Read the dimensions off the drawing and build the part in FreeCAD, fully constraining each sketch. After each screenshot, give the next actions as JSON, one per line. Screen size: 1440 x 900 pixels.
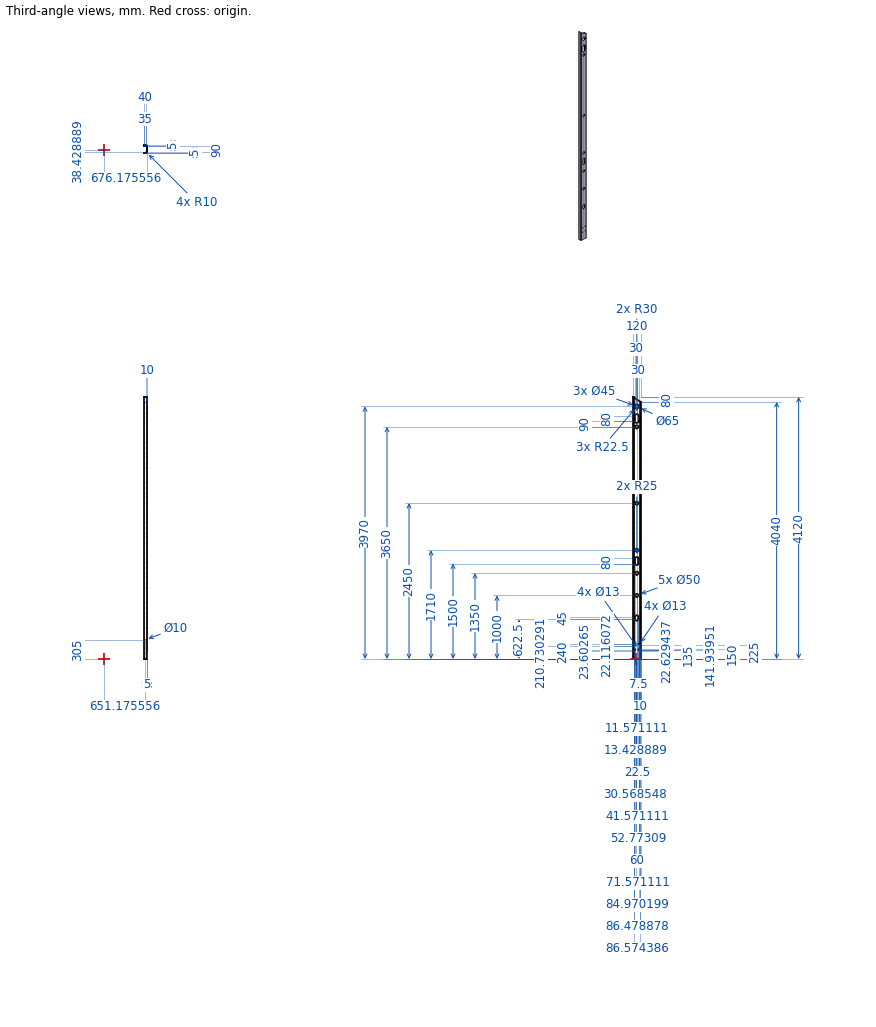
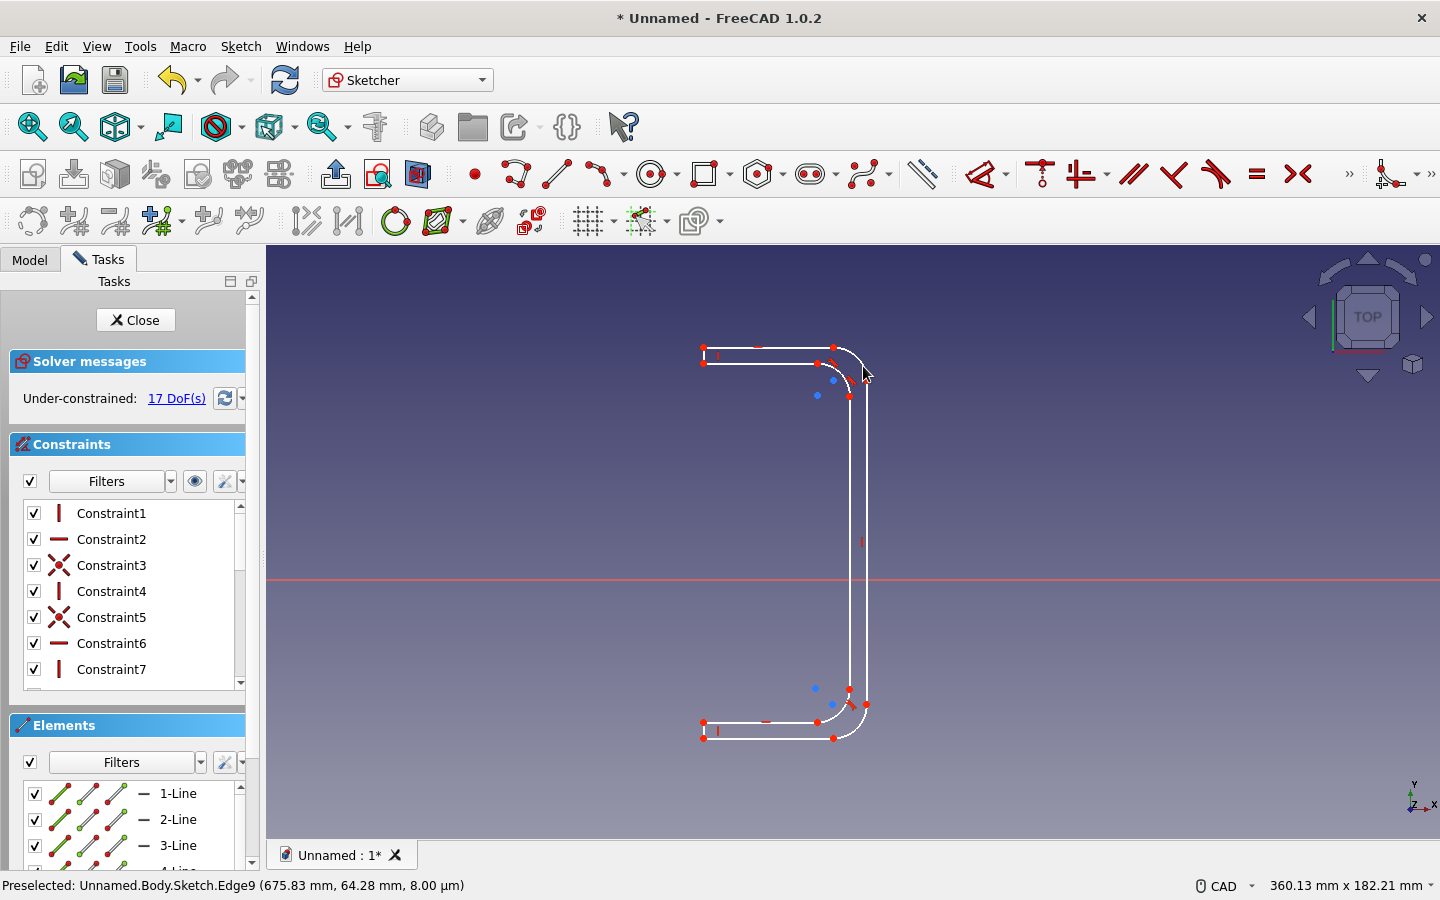
{"action": "left_click", "coordinate": [738, 364]}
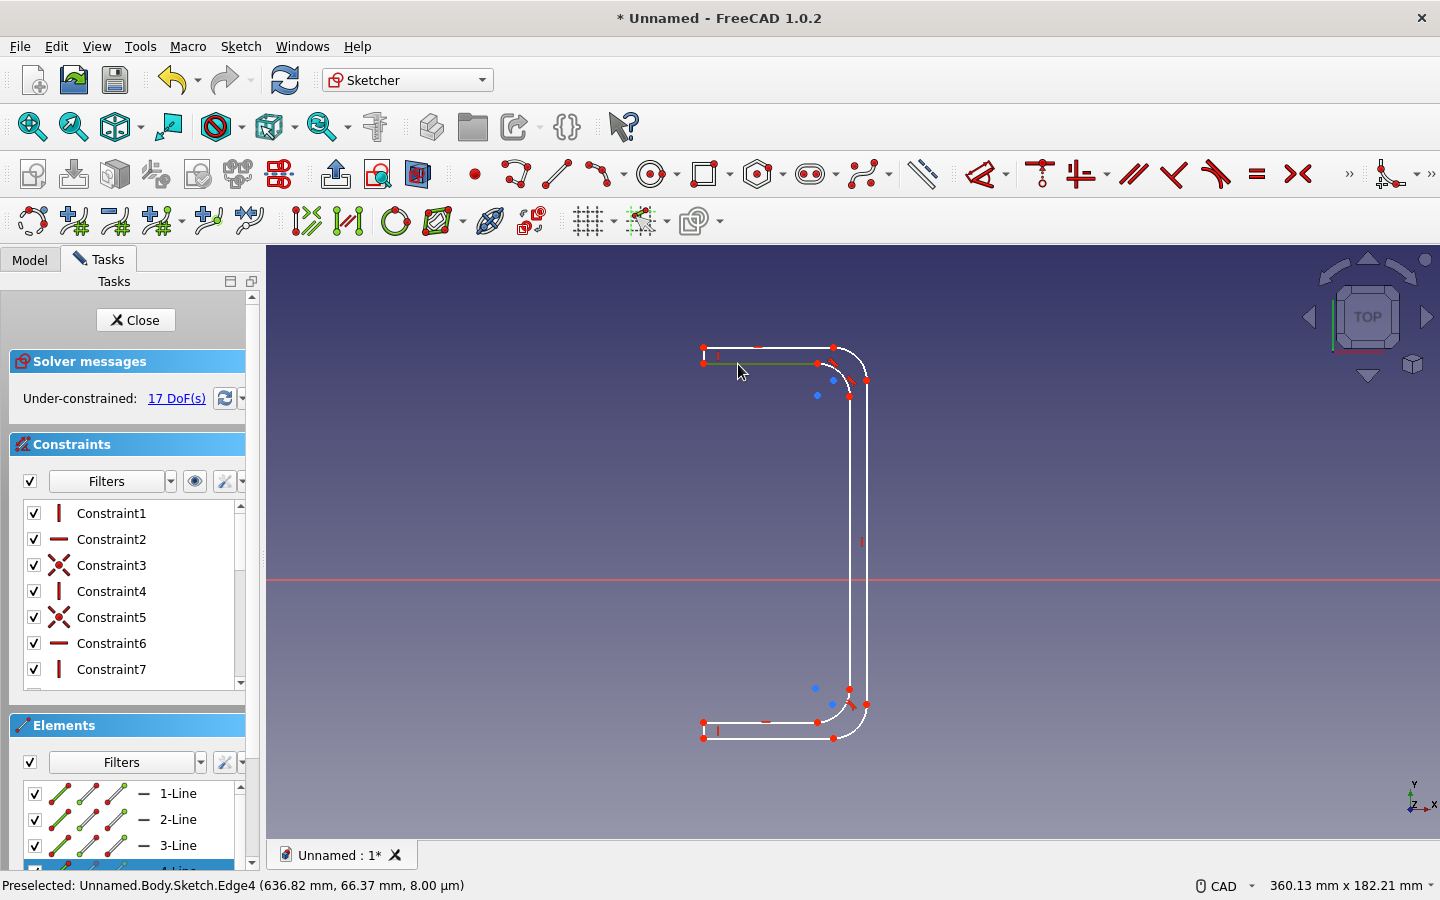
{"action": "left_click", "coordinate": [841, 373]}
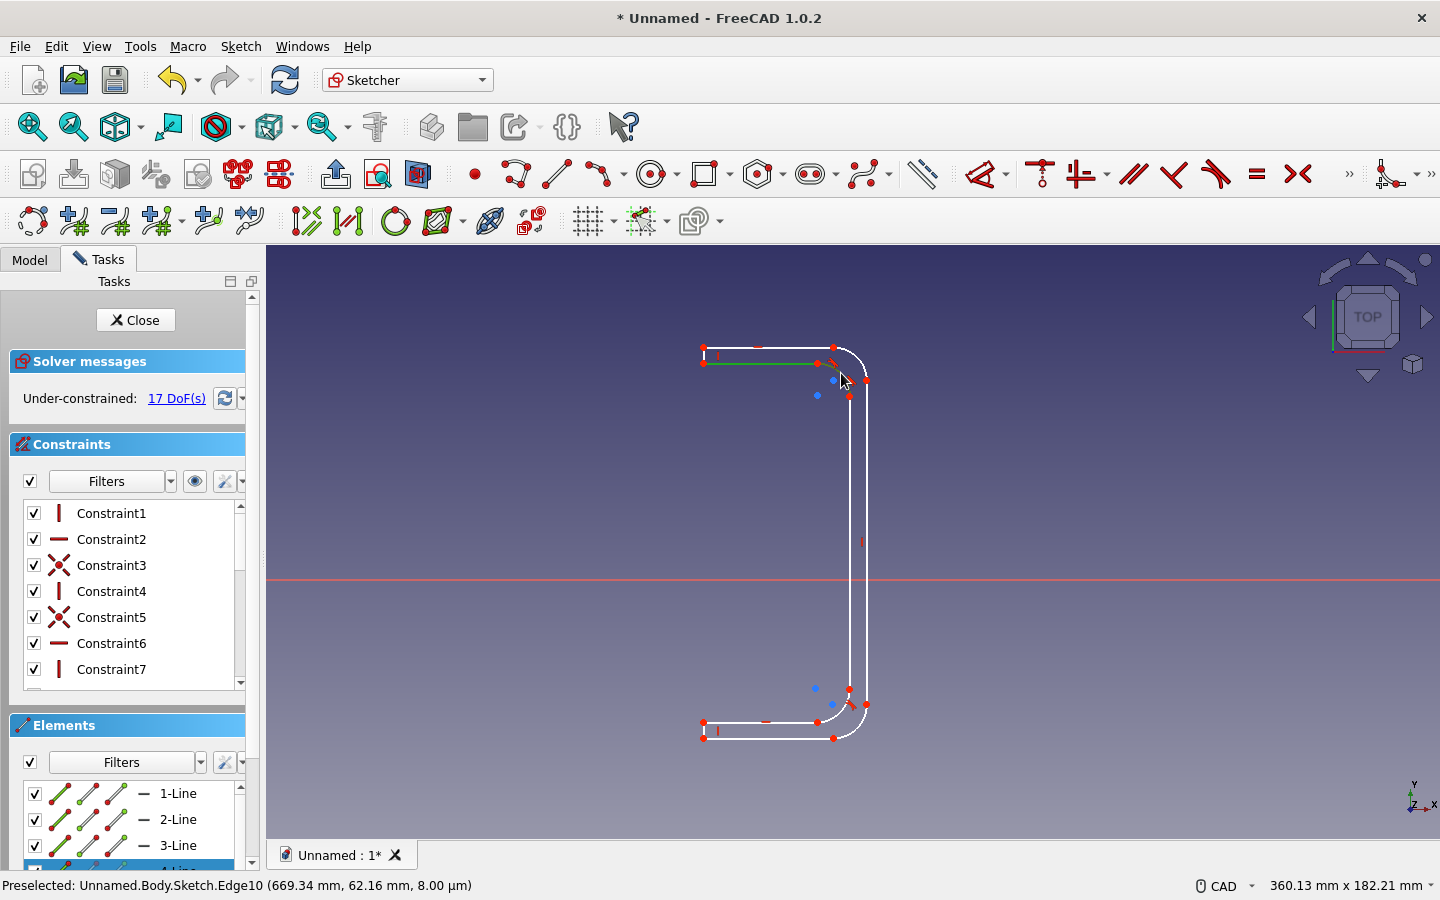
{"action": "key", "text": "t"}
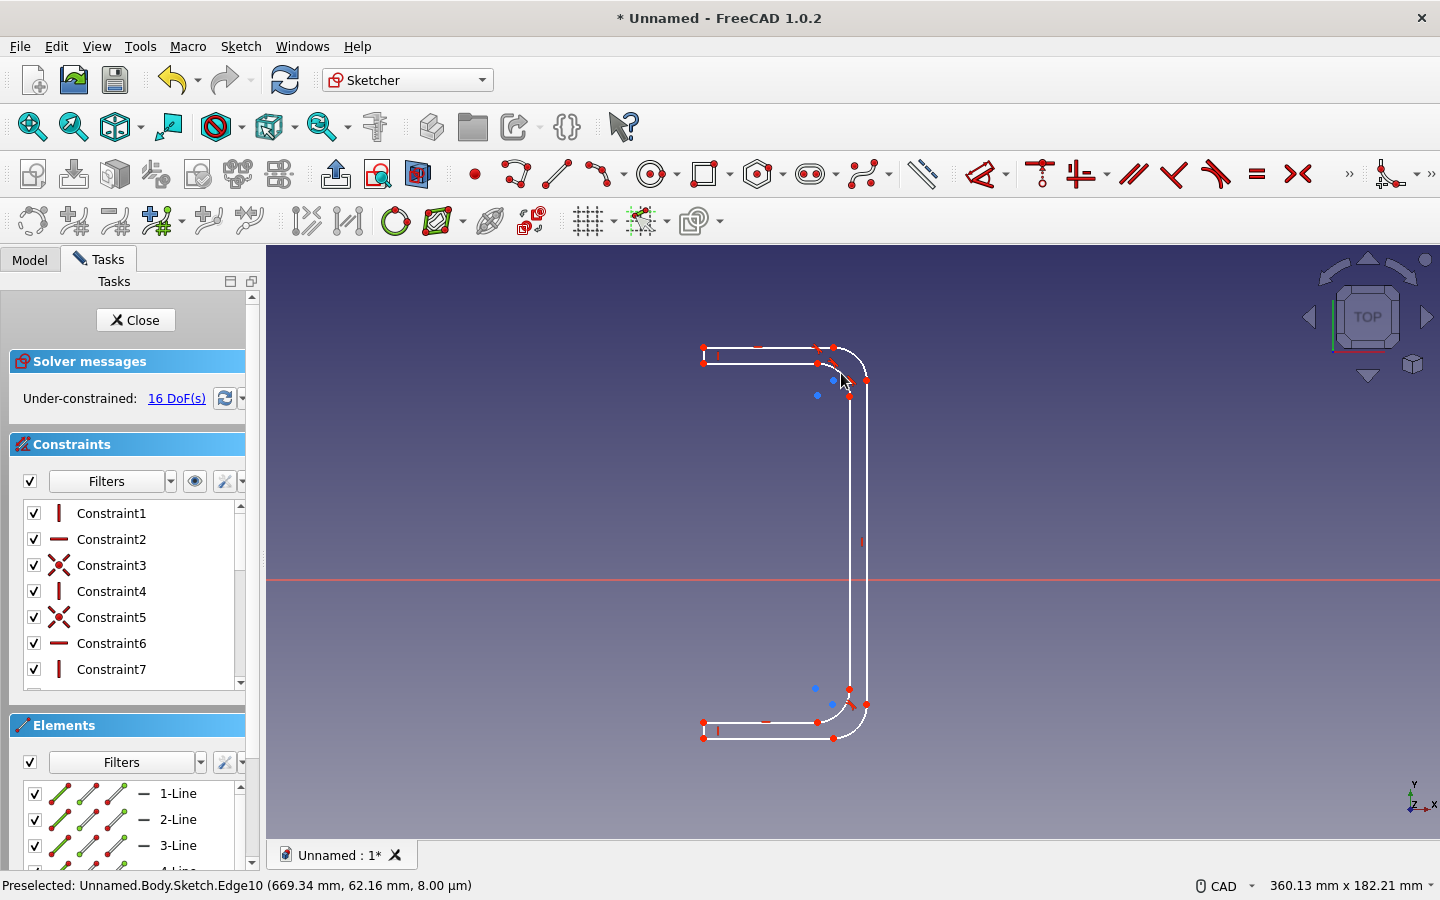
{"action": "left_click", "coordinate": [850, 485]}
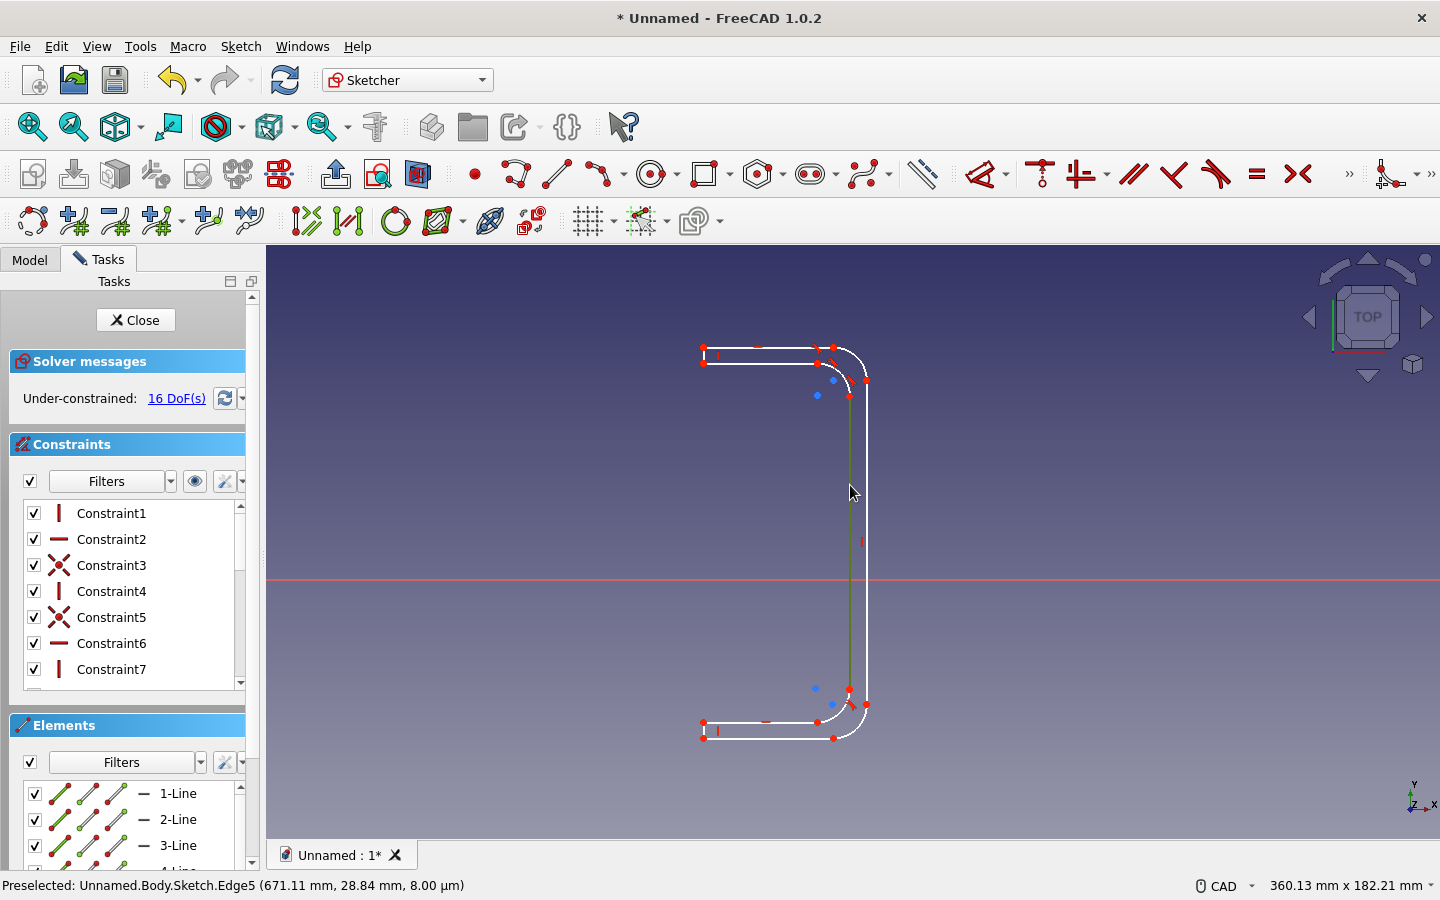
{"action": "left_click", "coordinate": [841, 373]}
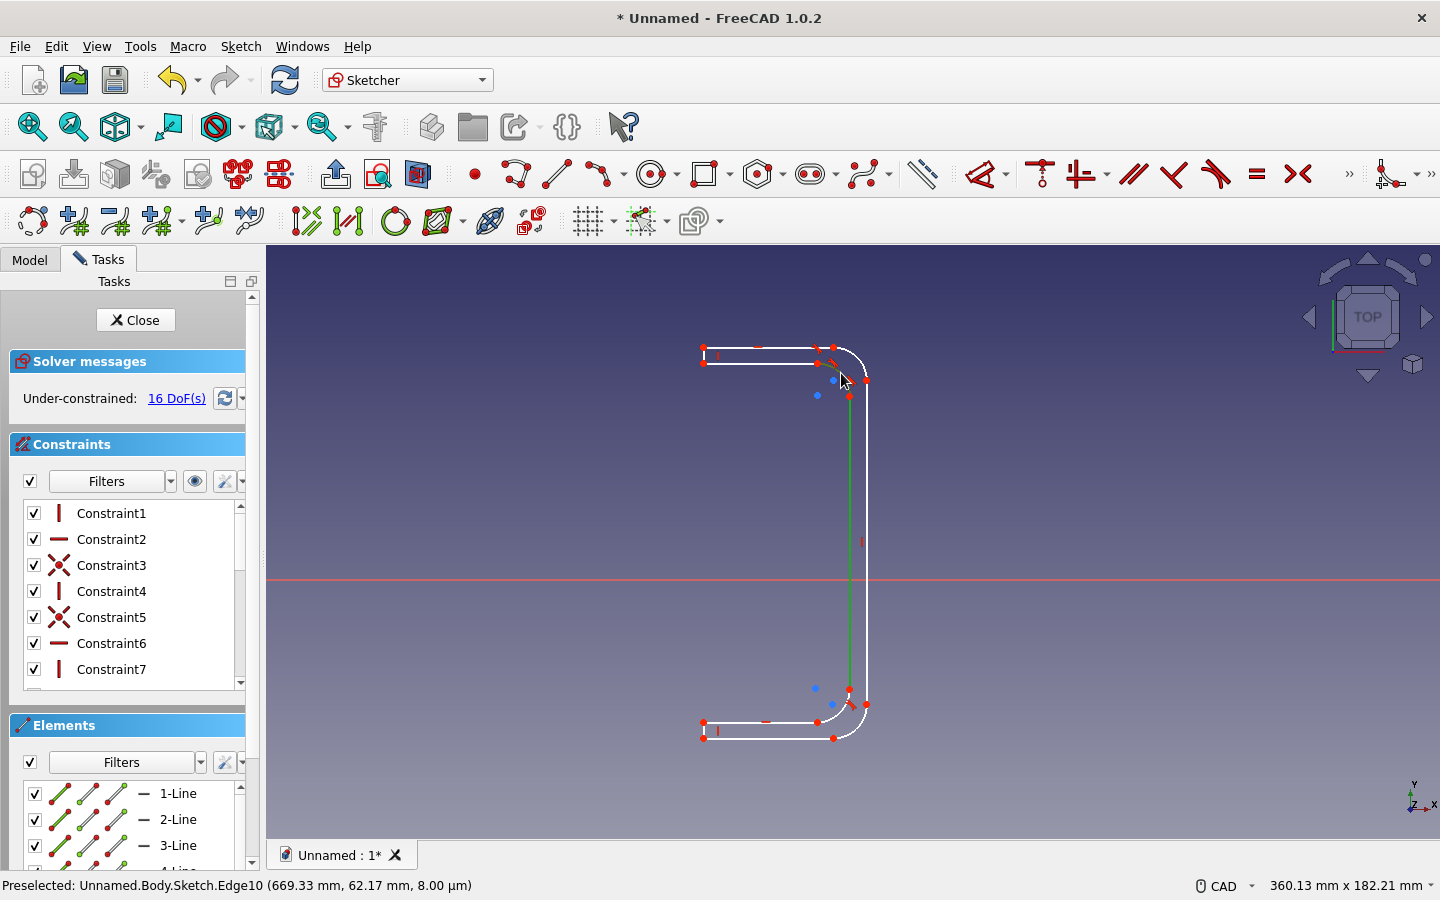
{"action": "key", "text": "t"}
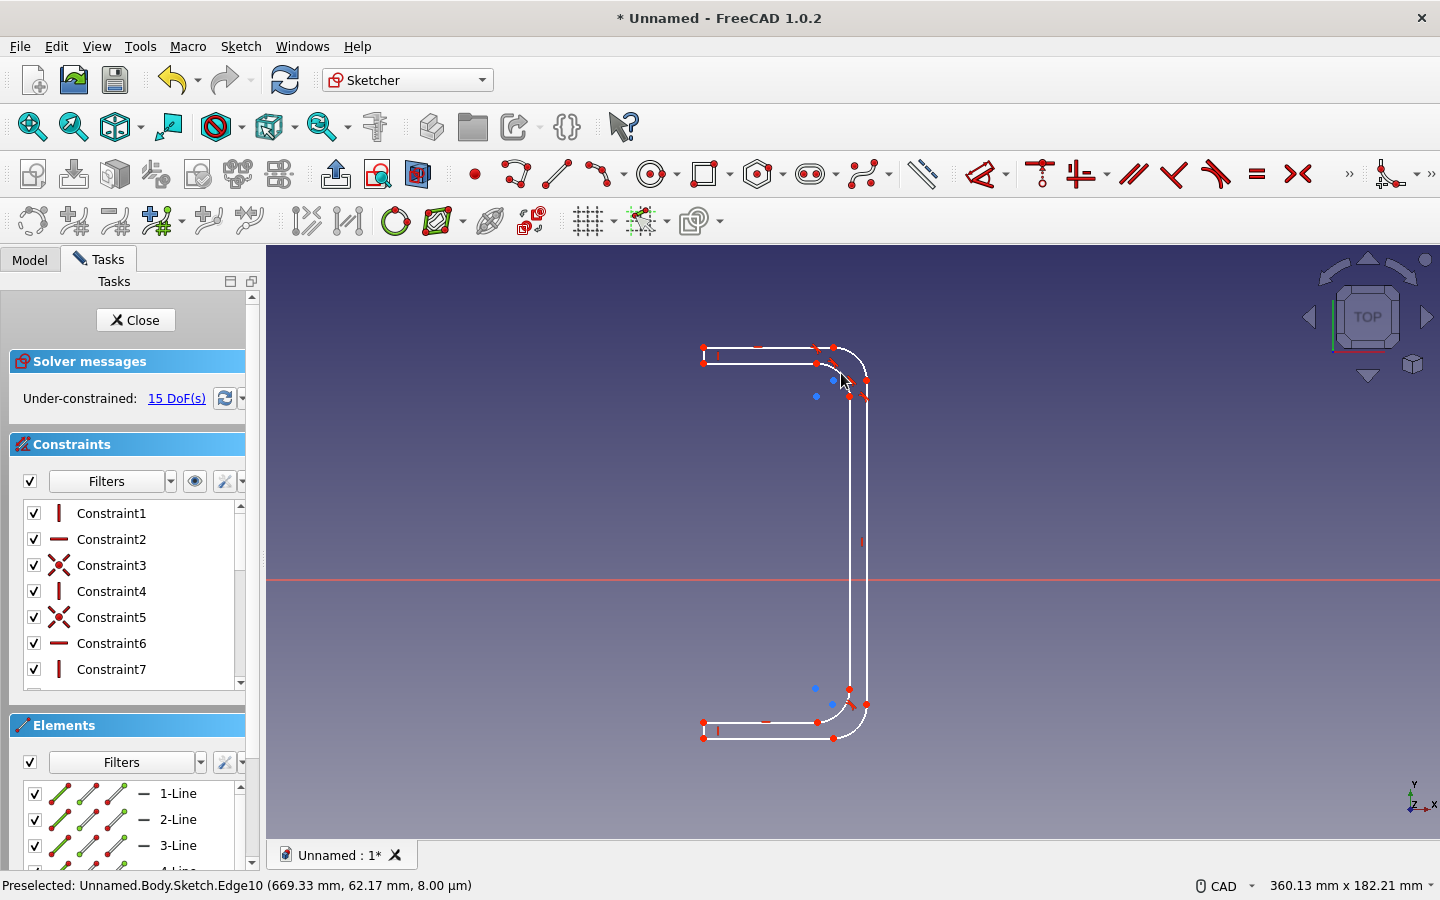
{"action": "left_click", "coordinate": [850, 485]}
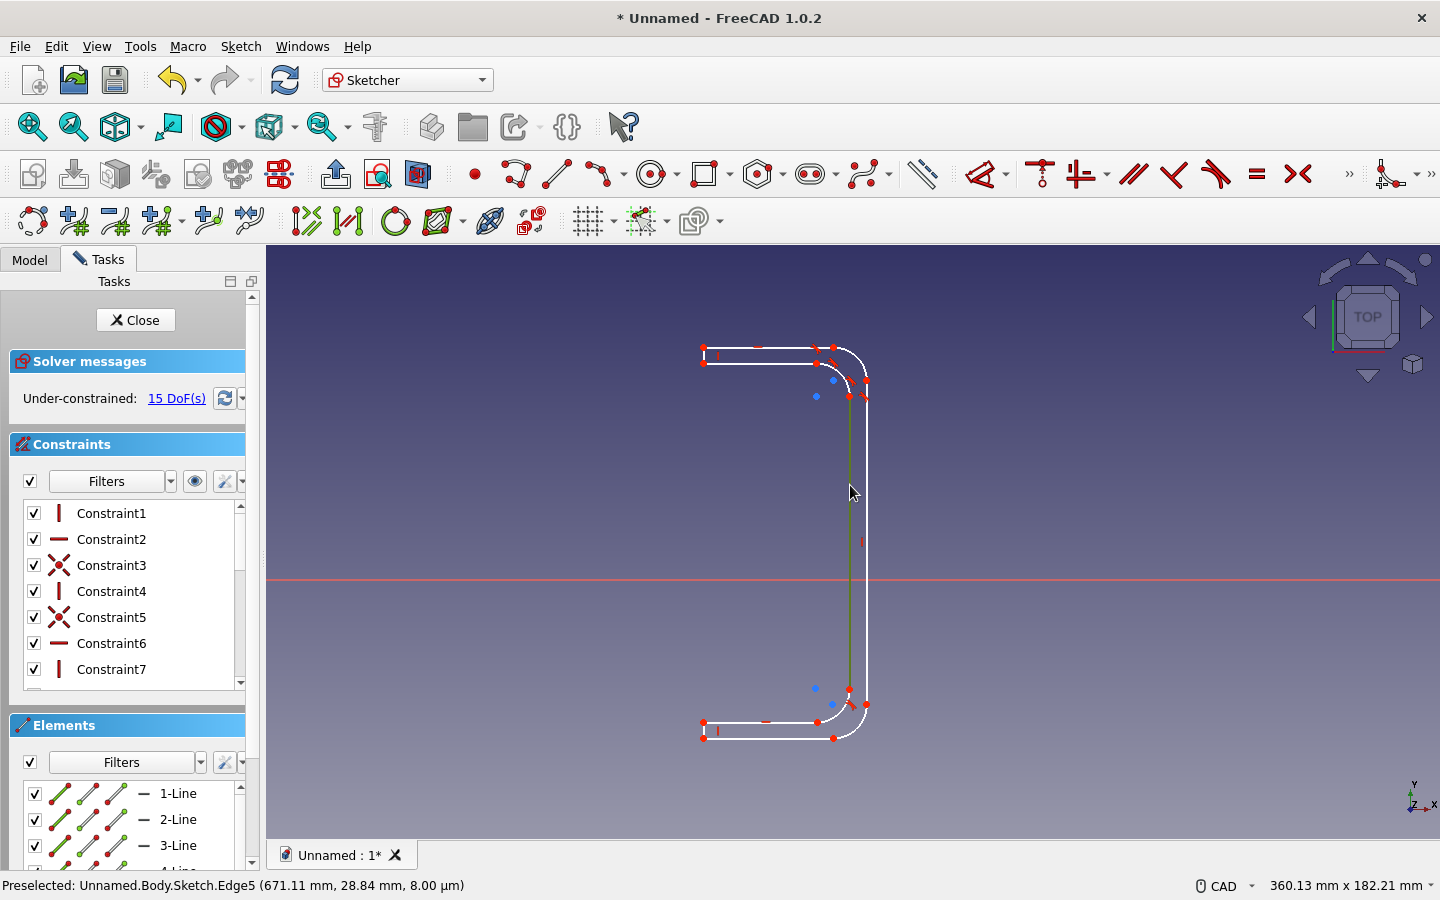
{"action": "left_click", "coordinate": [832, 719]}